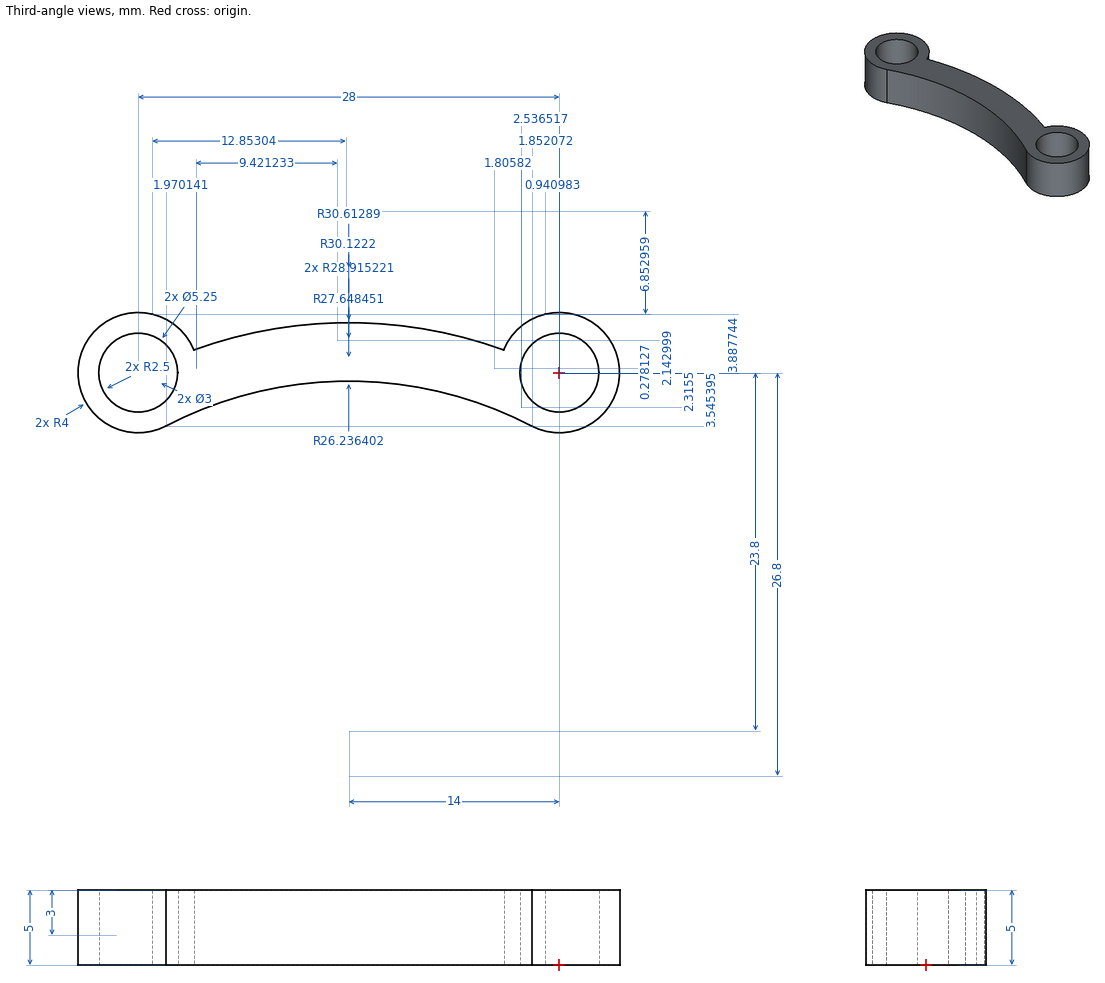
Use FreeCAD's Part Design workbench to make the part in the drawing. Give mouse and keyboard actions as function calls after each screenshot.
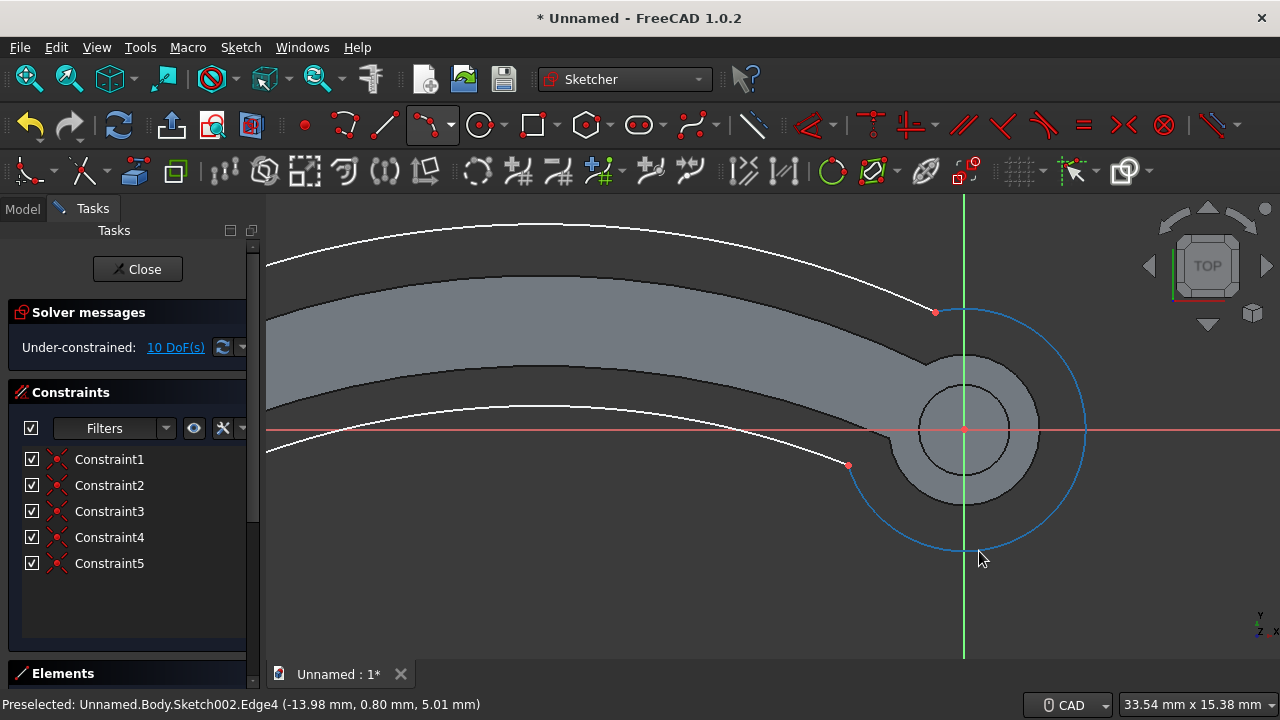
click(979, 550)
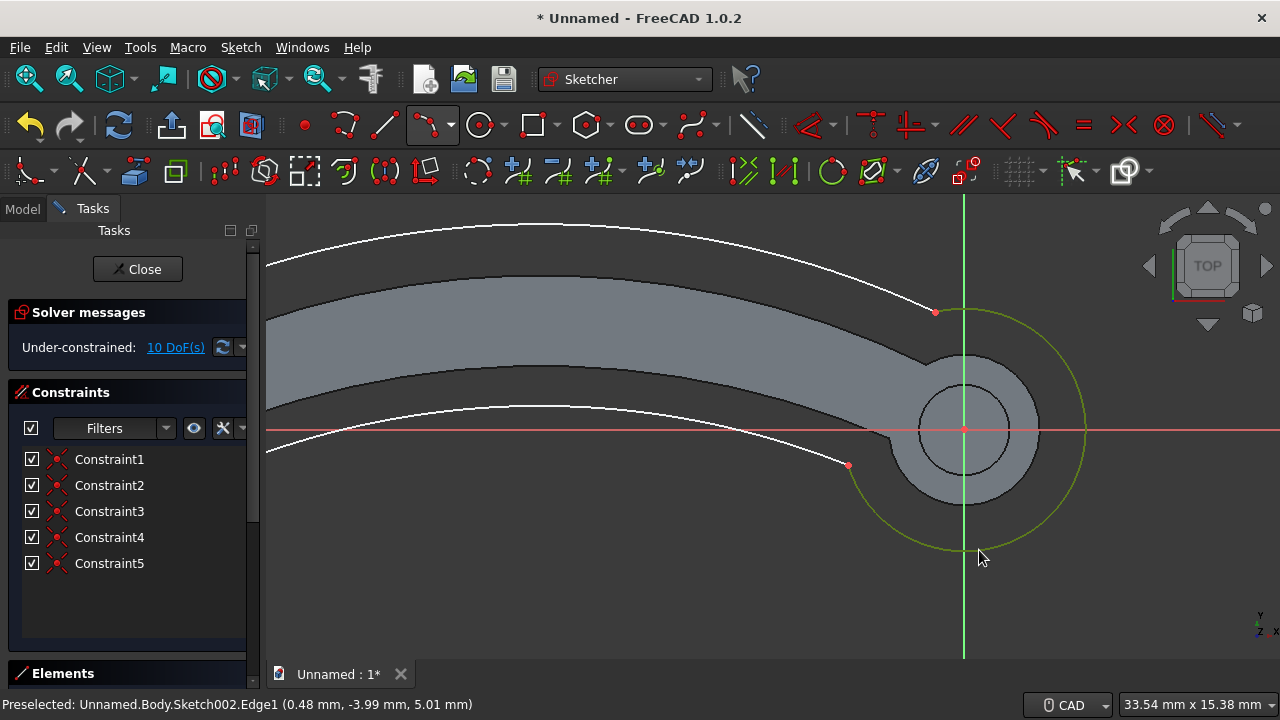
scroll(903, 510, down, 3)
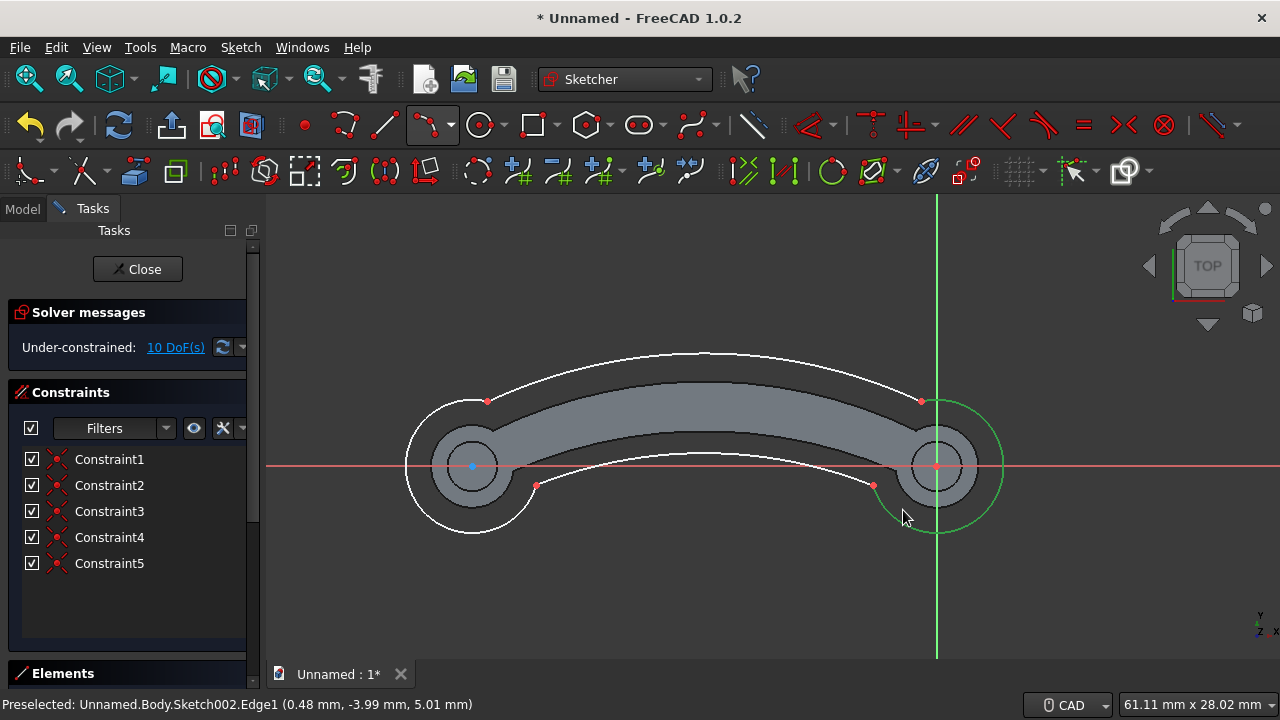
click(411, 440)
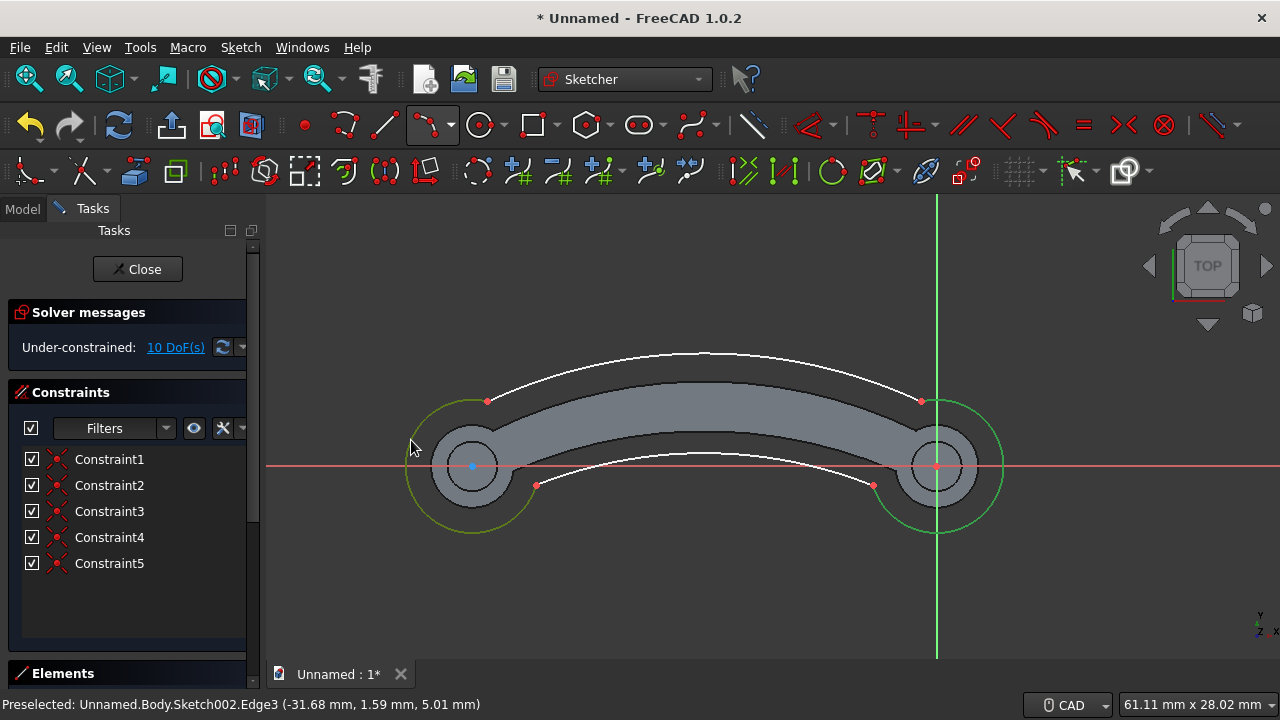
click(1084, 126)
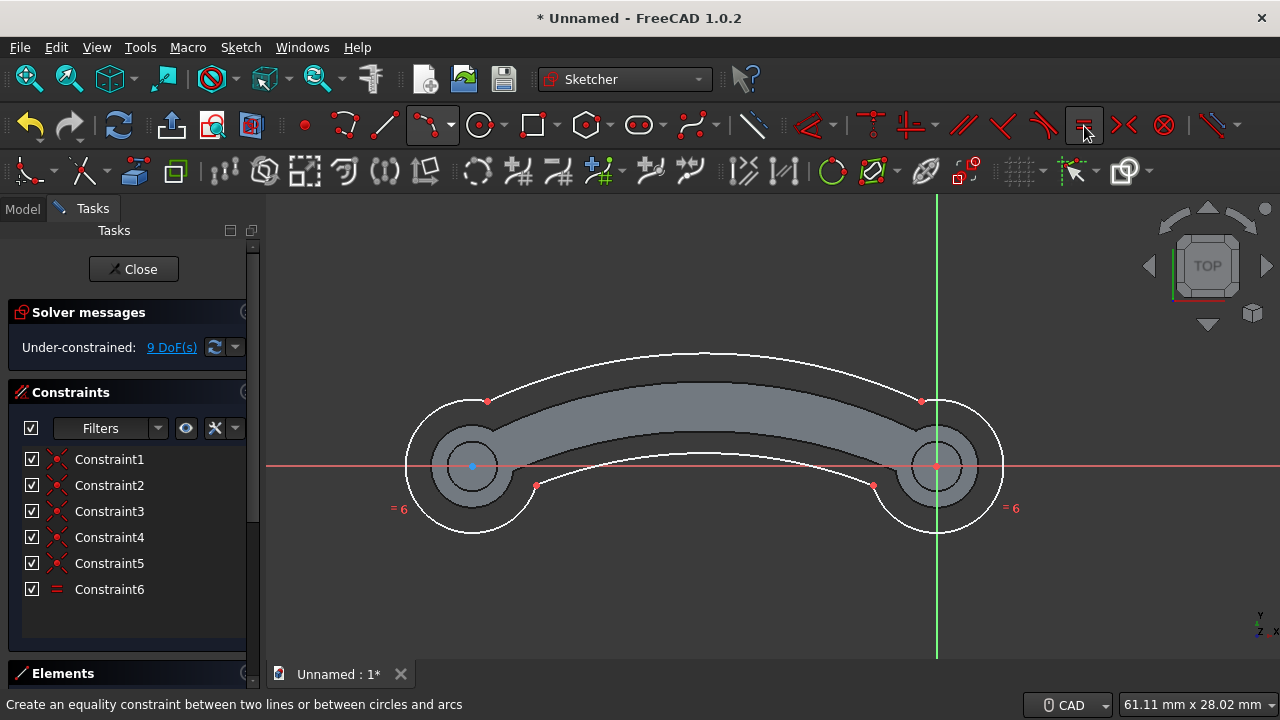
click(472, 466)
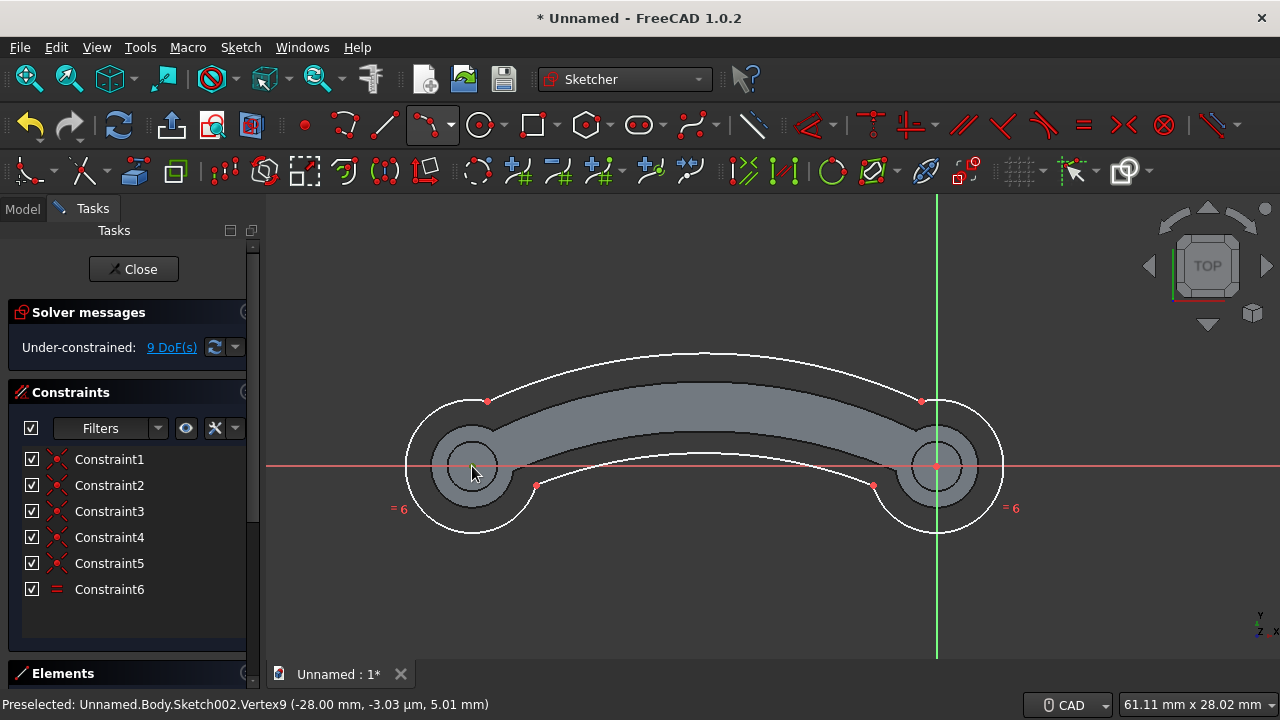
click(353, 466)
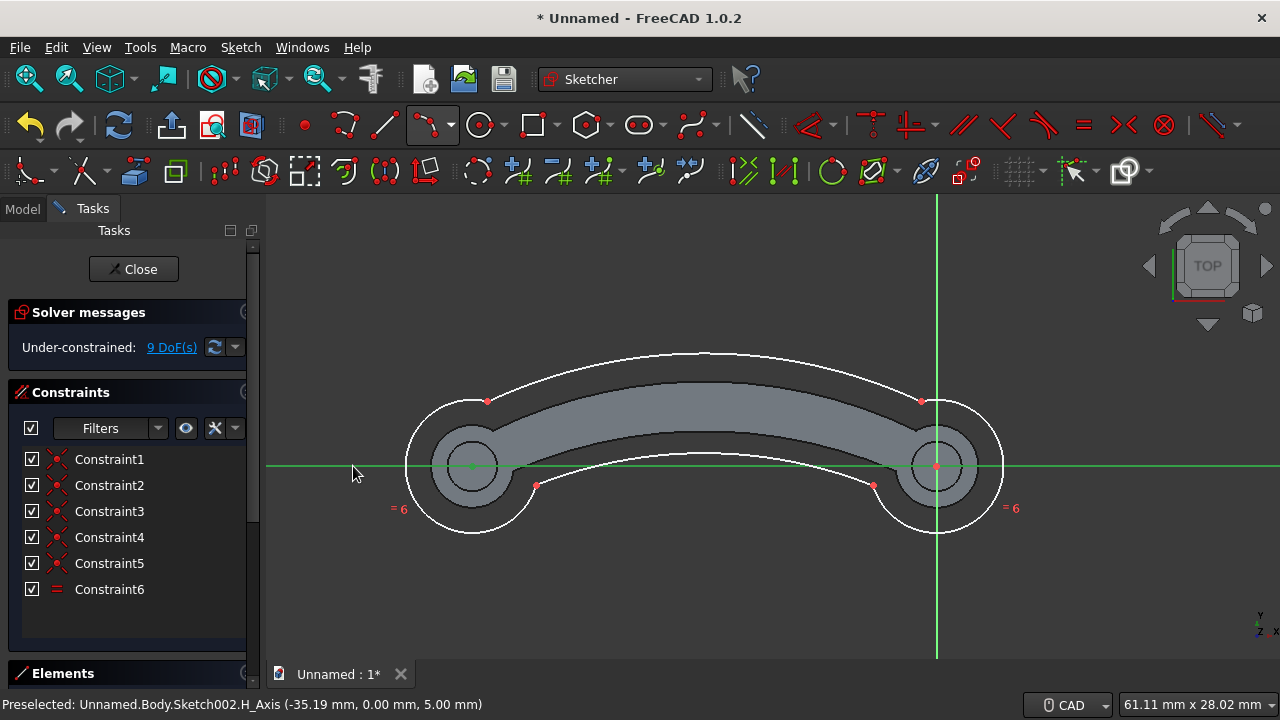
click(872, 126)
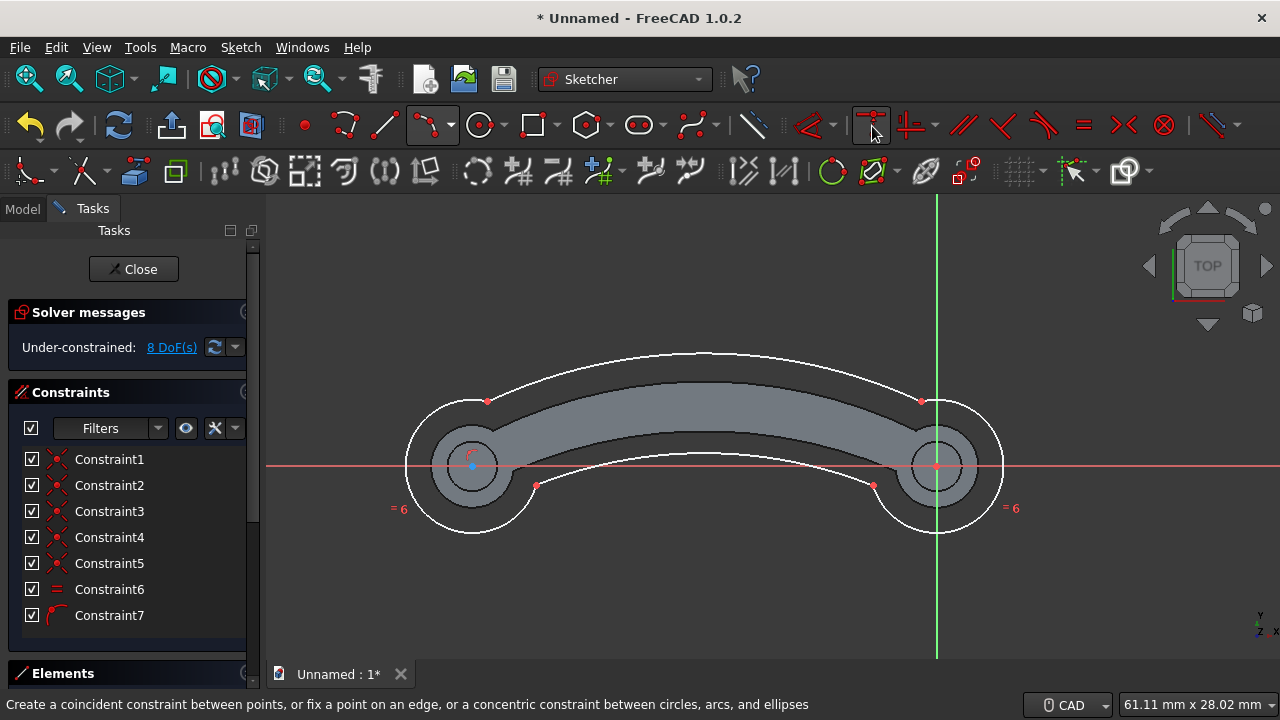
key(d)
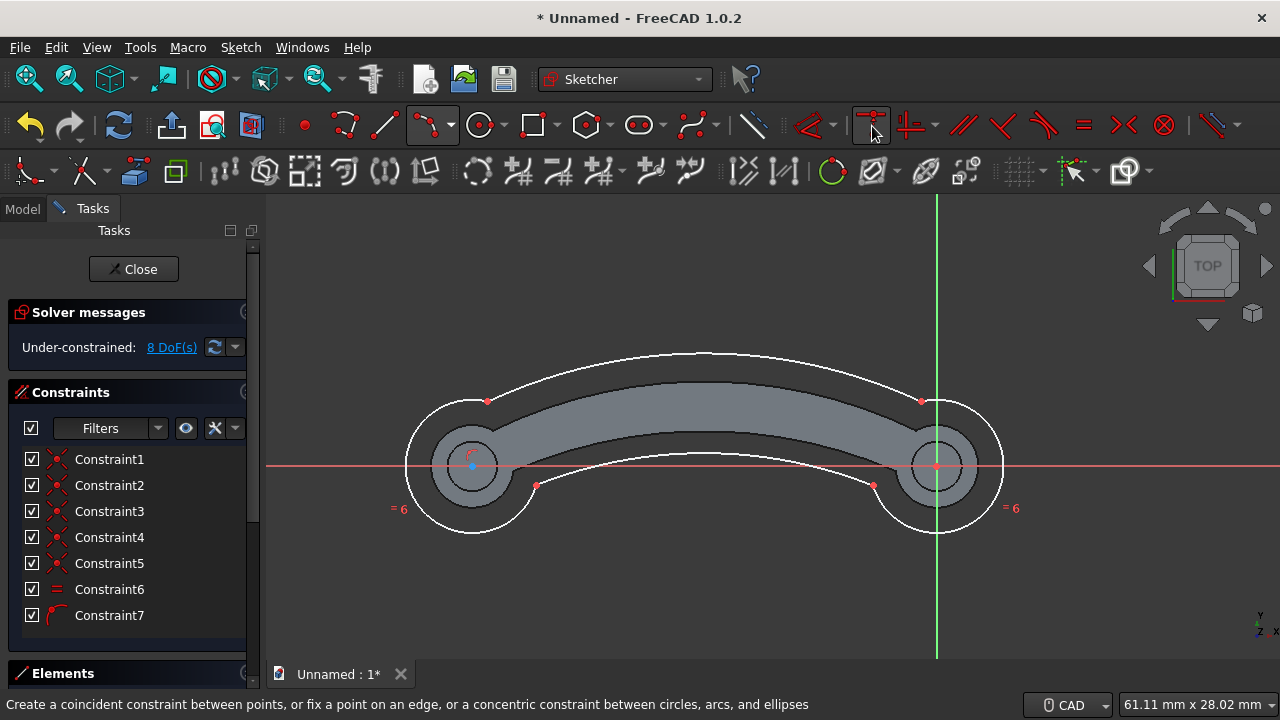
click(998, 440)
click(1027, 427)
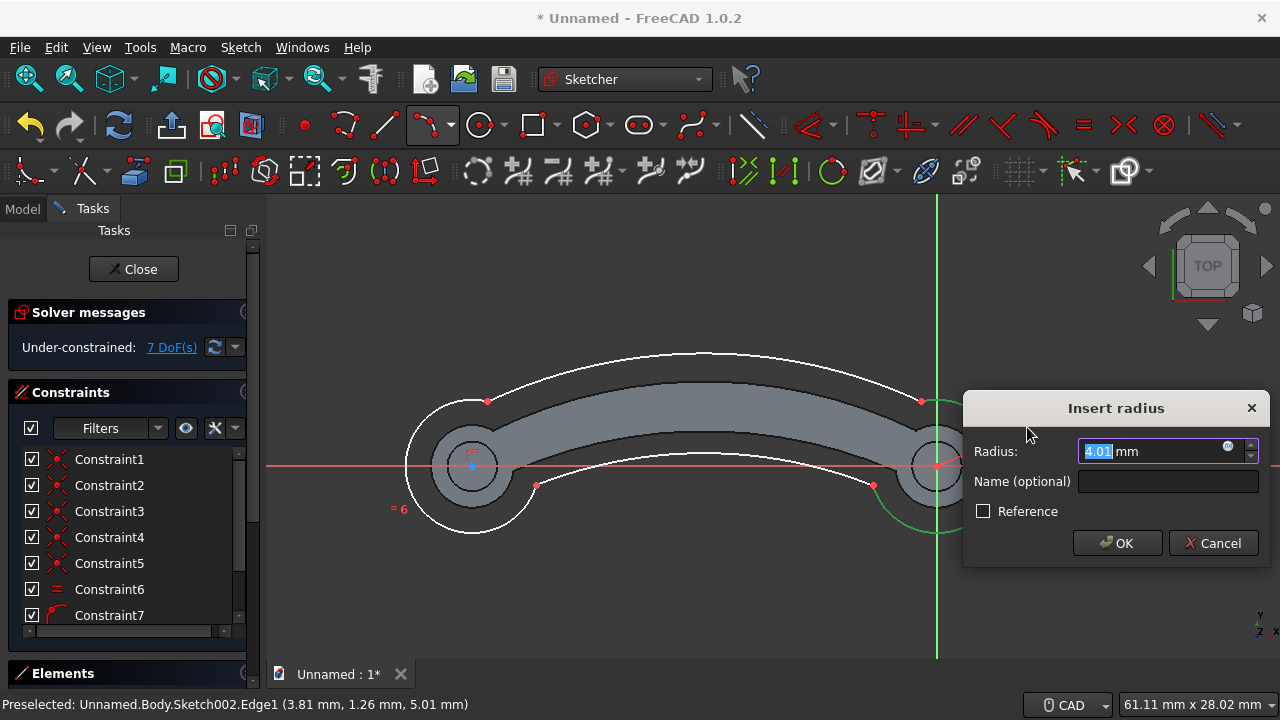
text(4)
key(Return)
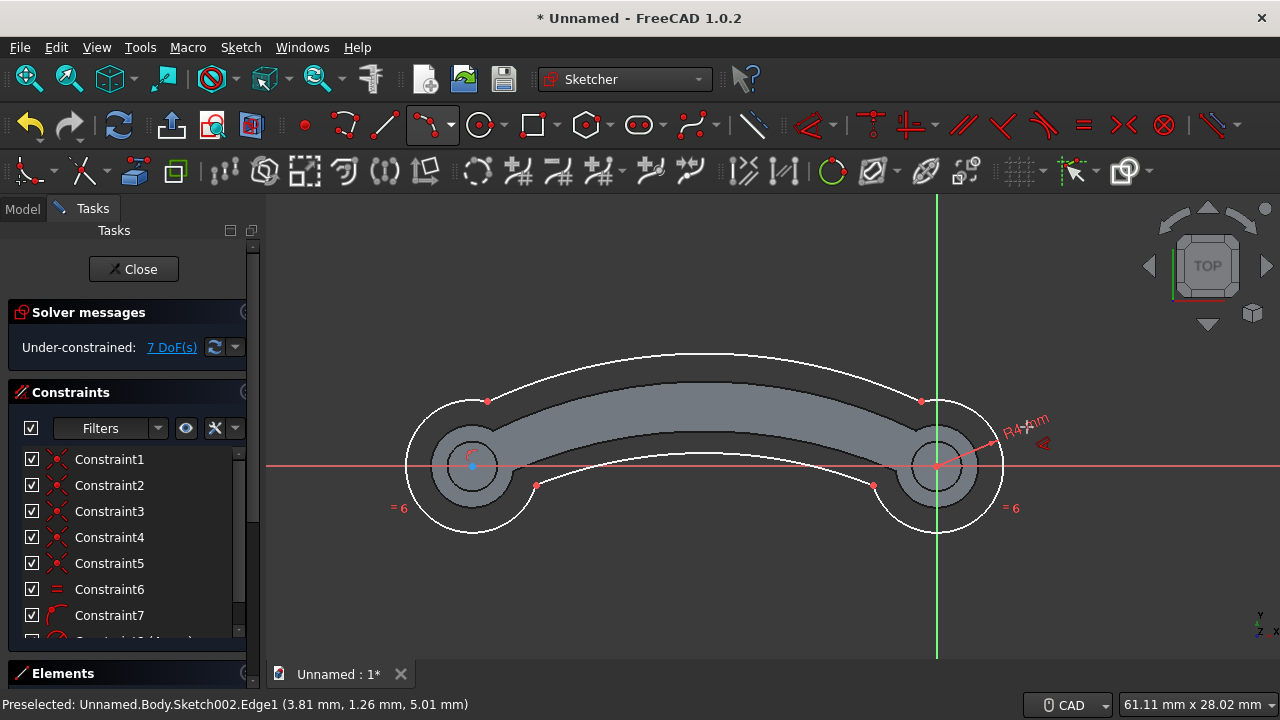
click(794, 361)
click(800, 329)